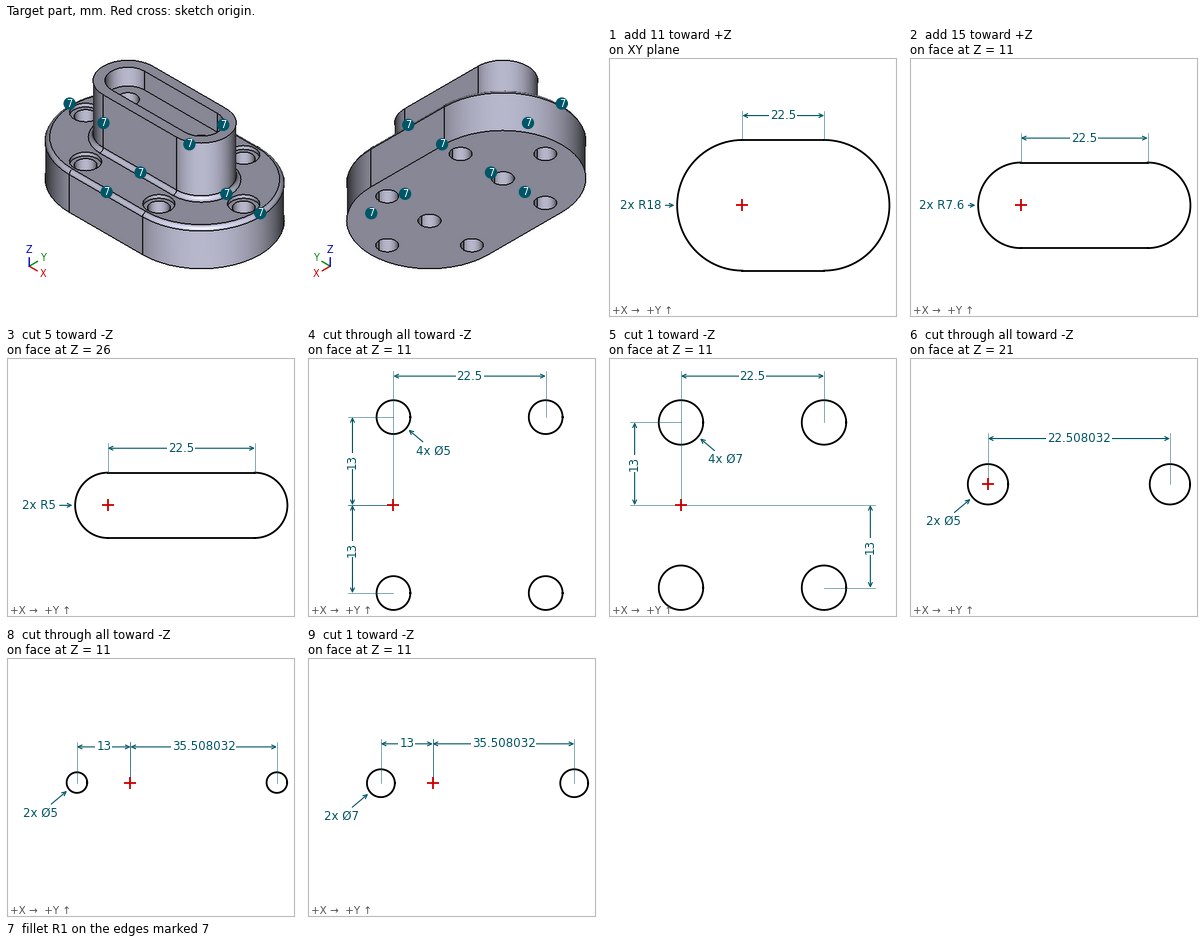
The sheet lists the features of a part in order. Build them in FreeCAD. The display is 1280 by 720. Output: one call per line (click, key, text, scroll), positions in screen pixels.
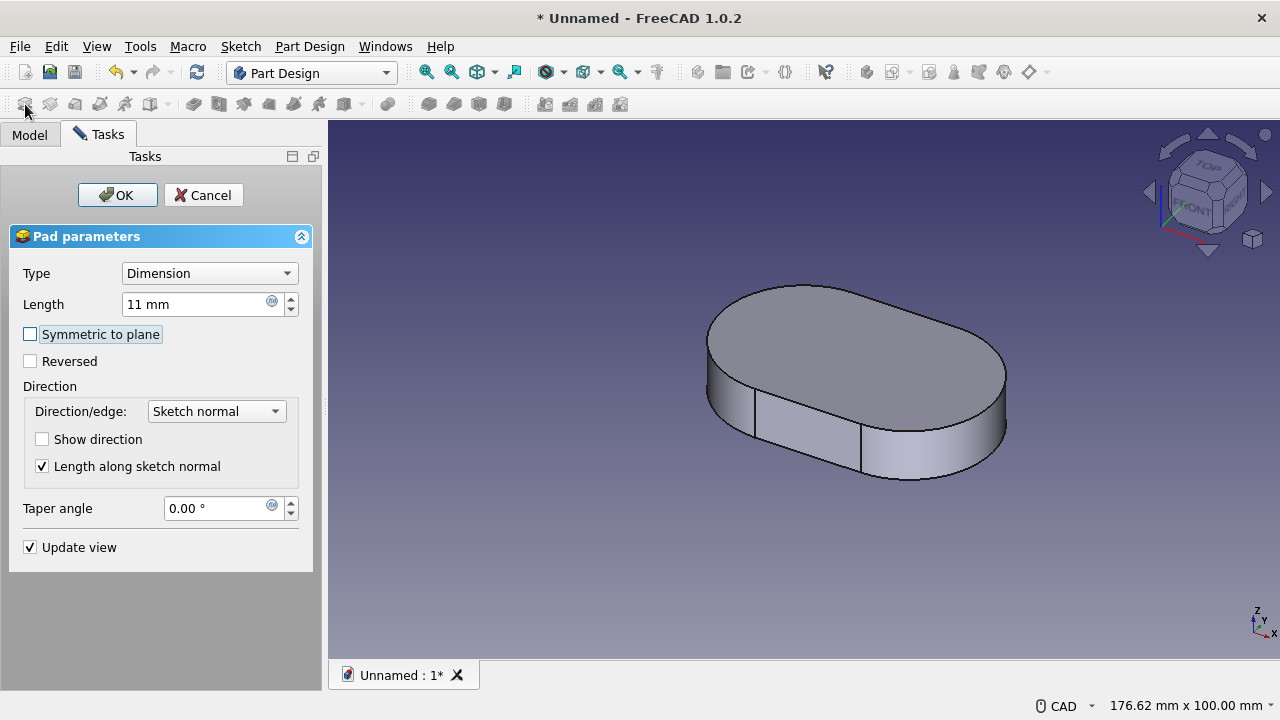
click(118, 195)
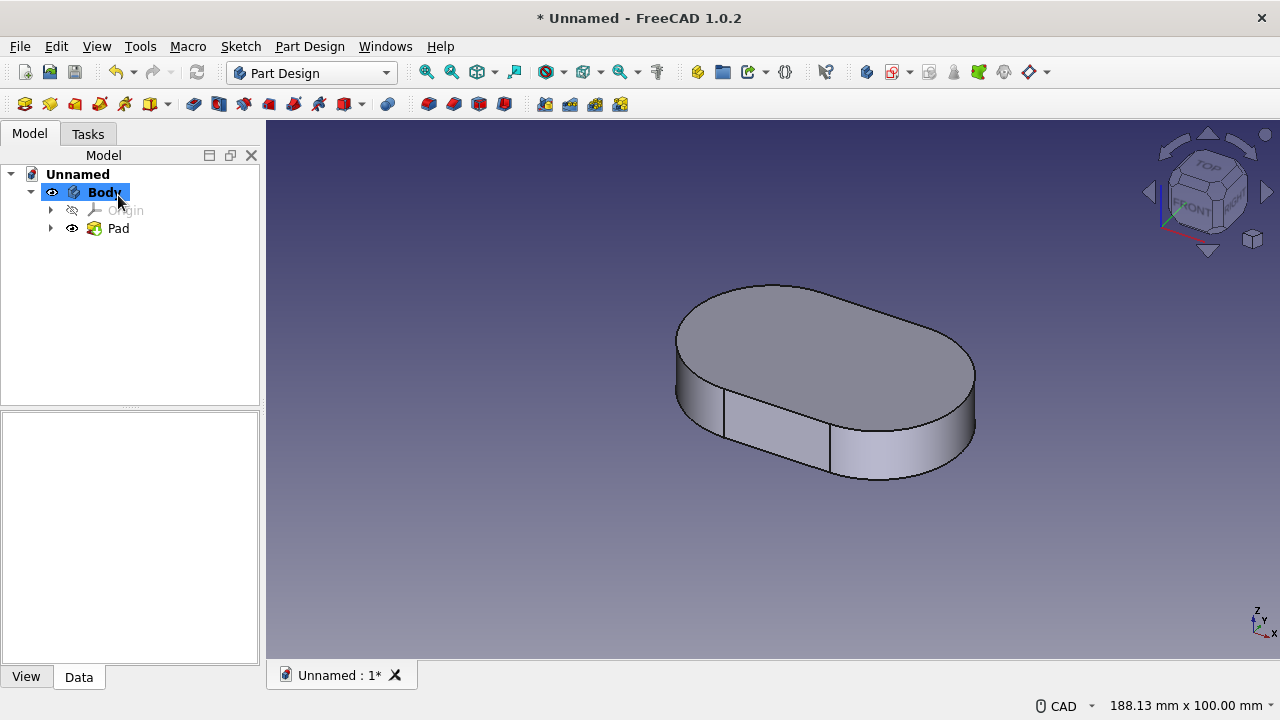
click(427, 72)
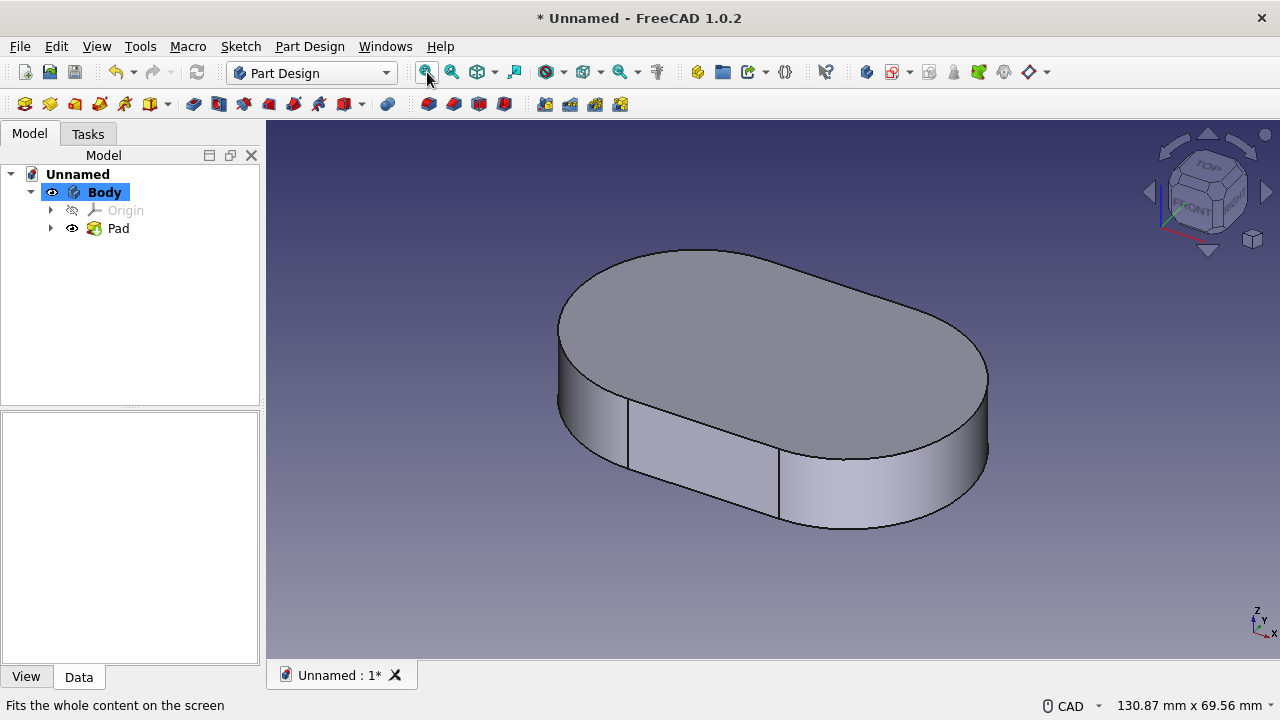
click(829, 372)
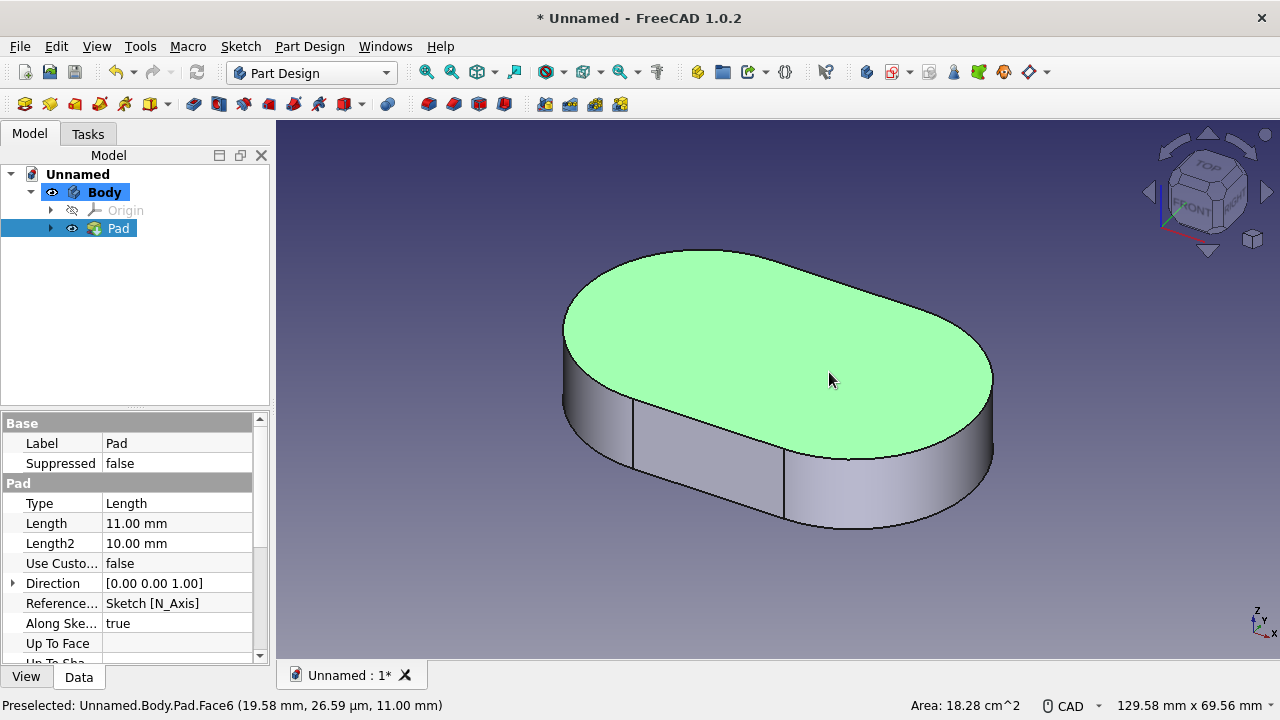
click(892, 72)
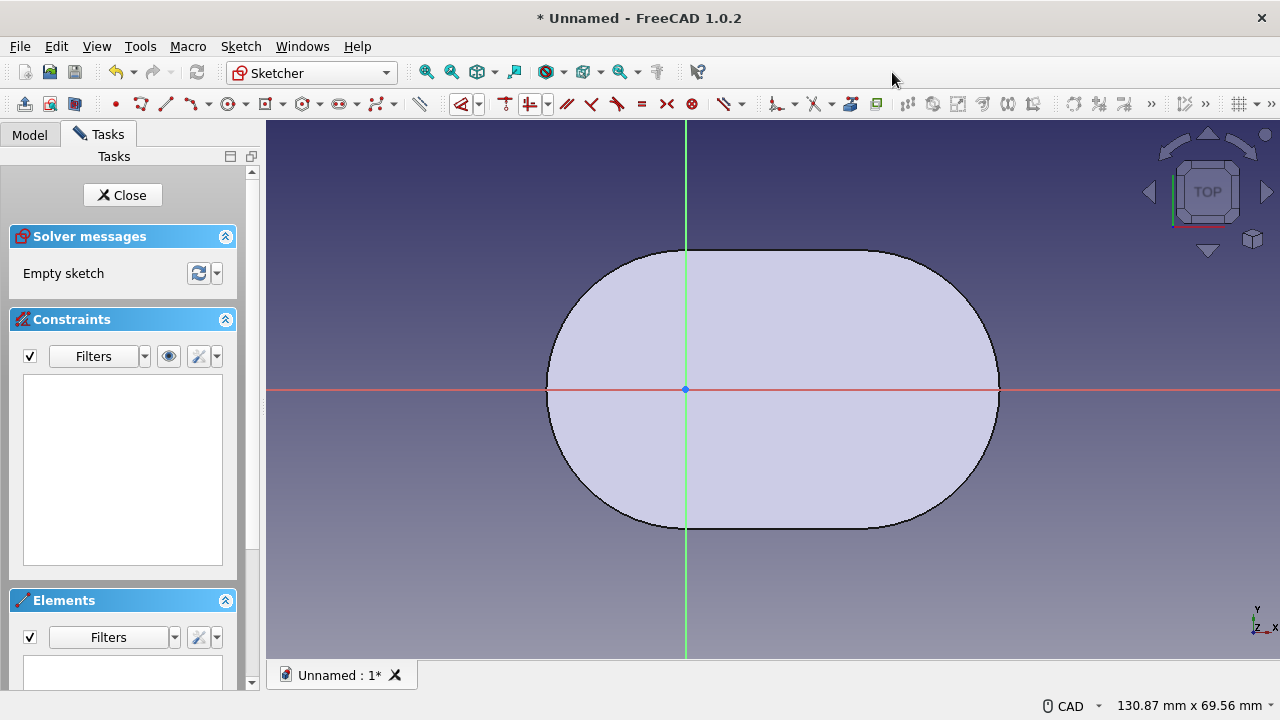
scroll(856, 389, up, 3)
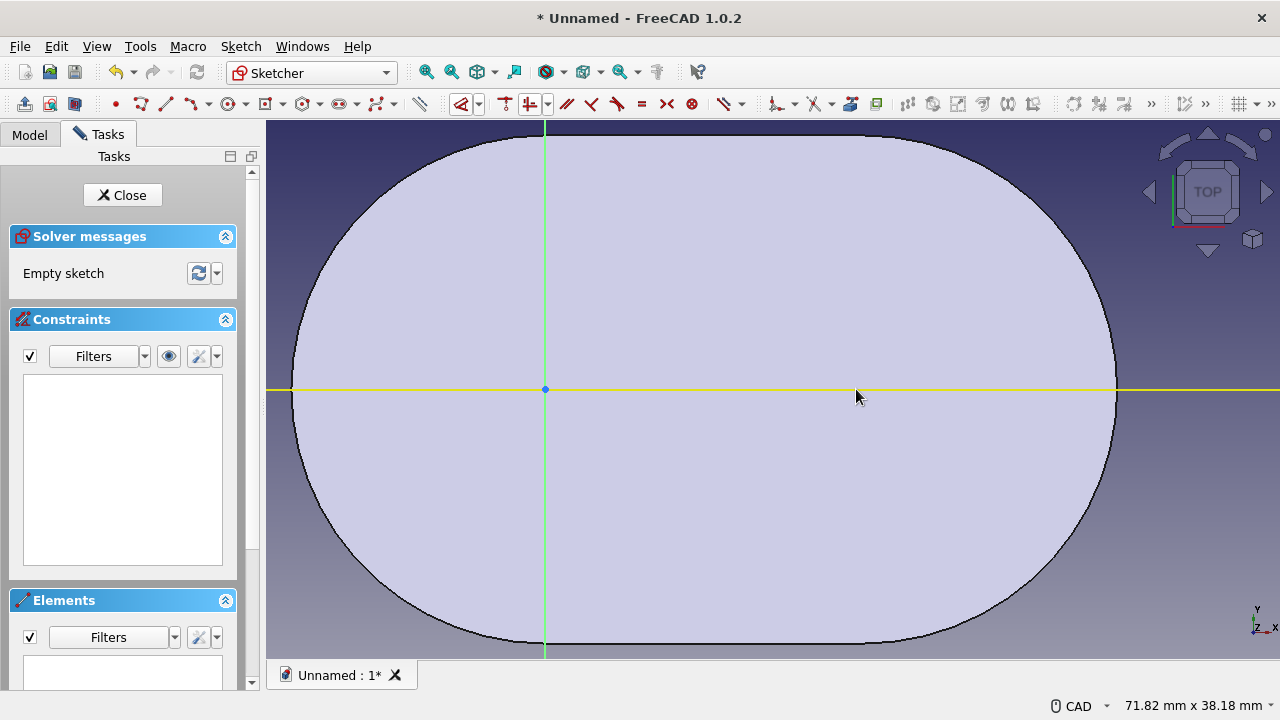
key(g)
key(s)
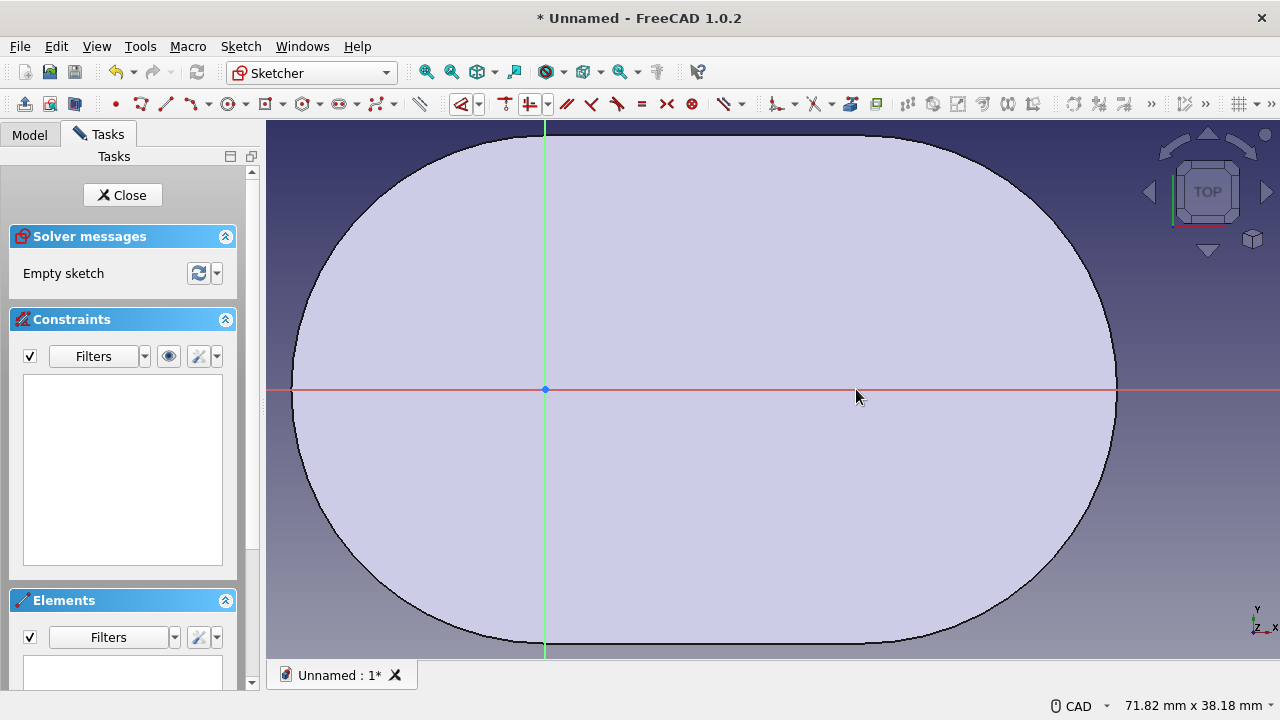
click(545, 390)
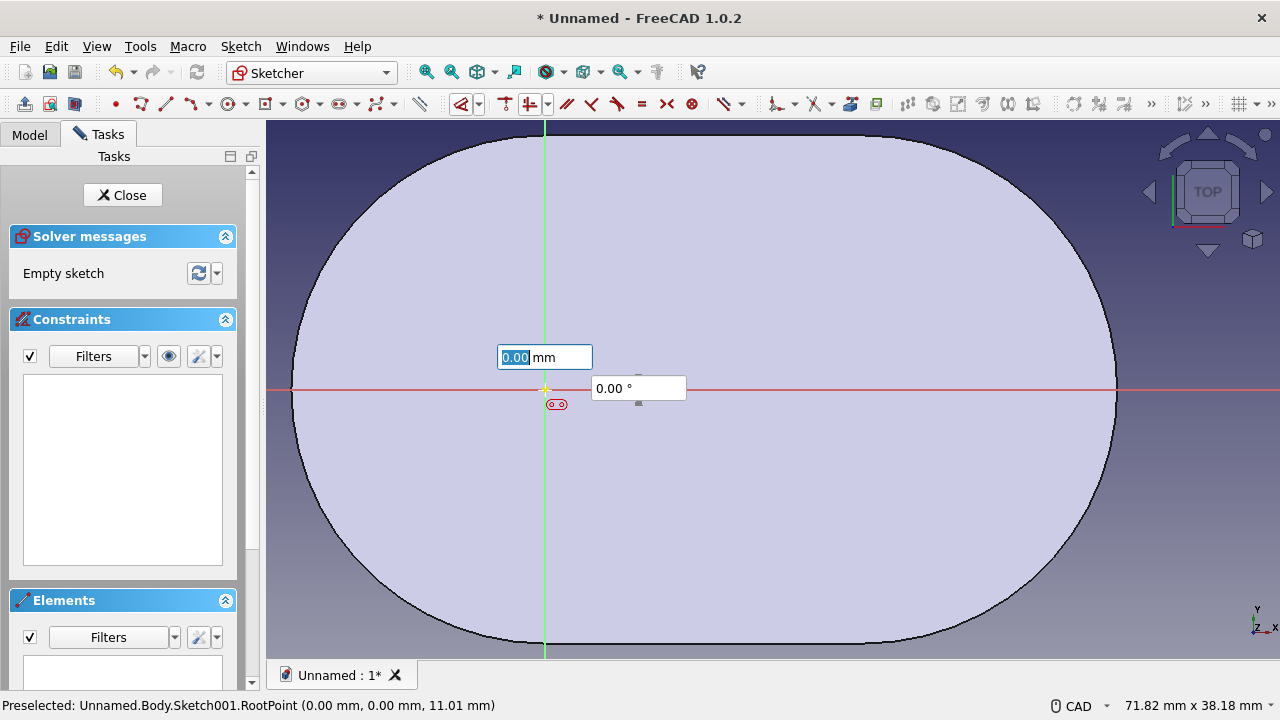
click(863, 380)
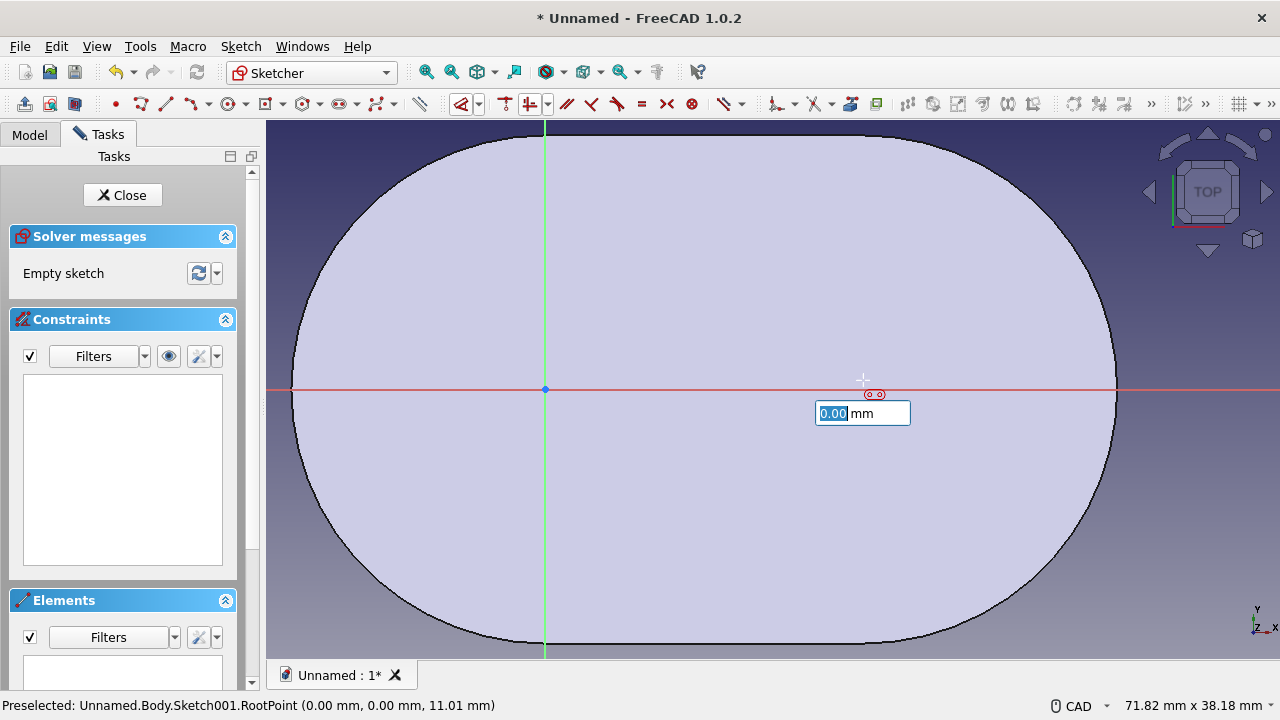
click(704, 282)
key(Escape)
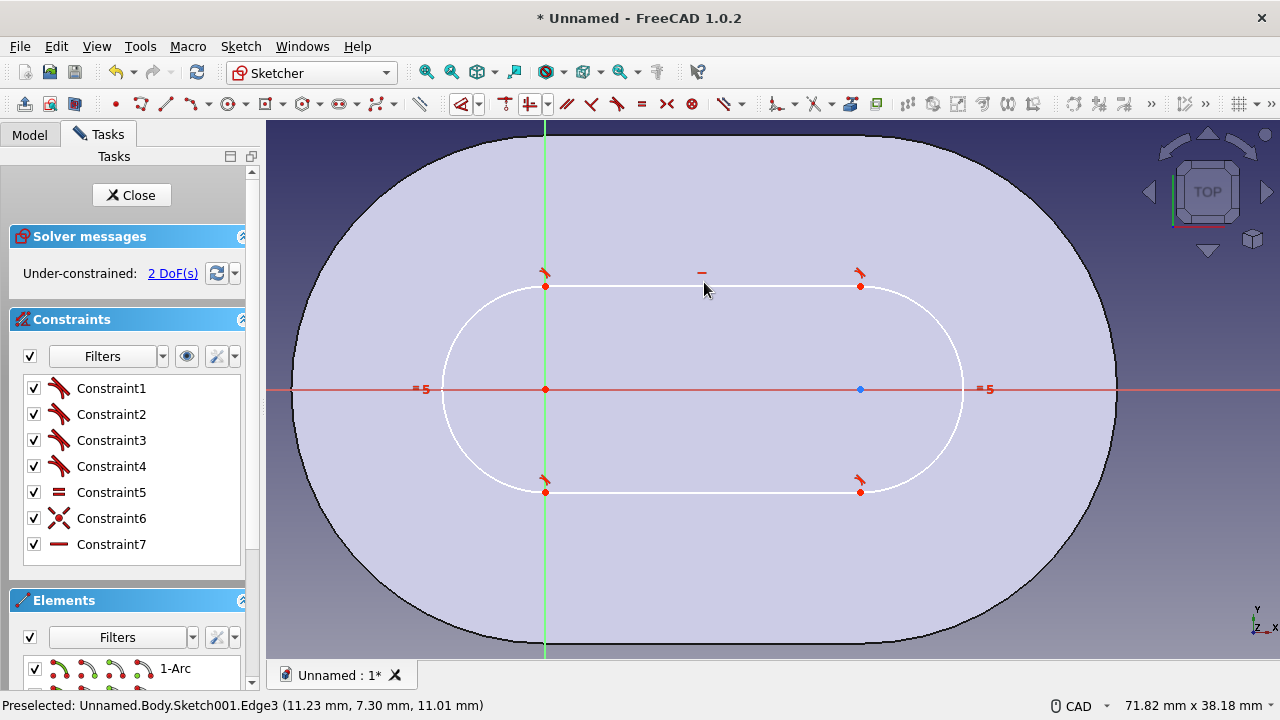
click(462, 329)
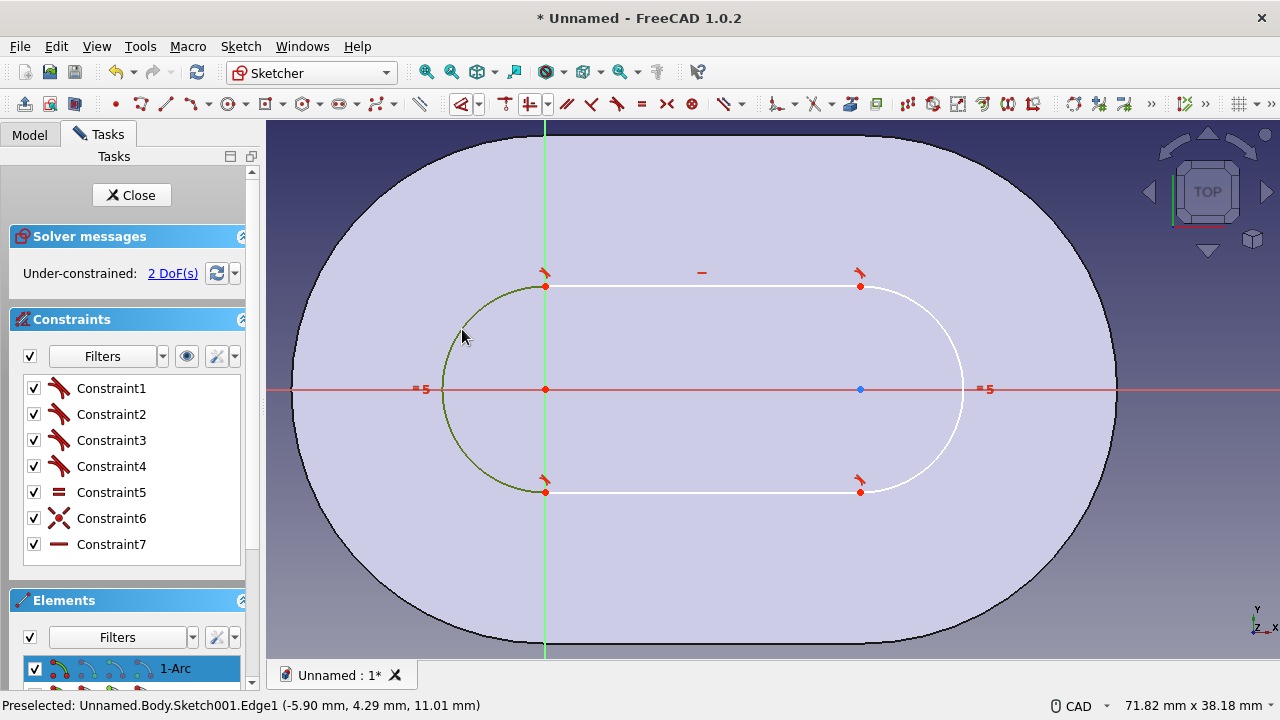
key(k)
key(r)